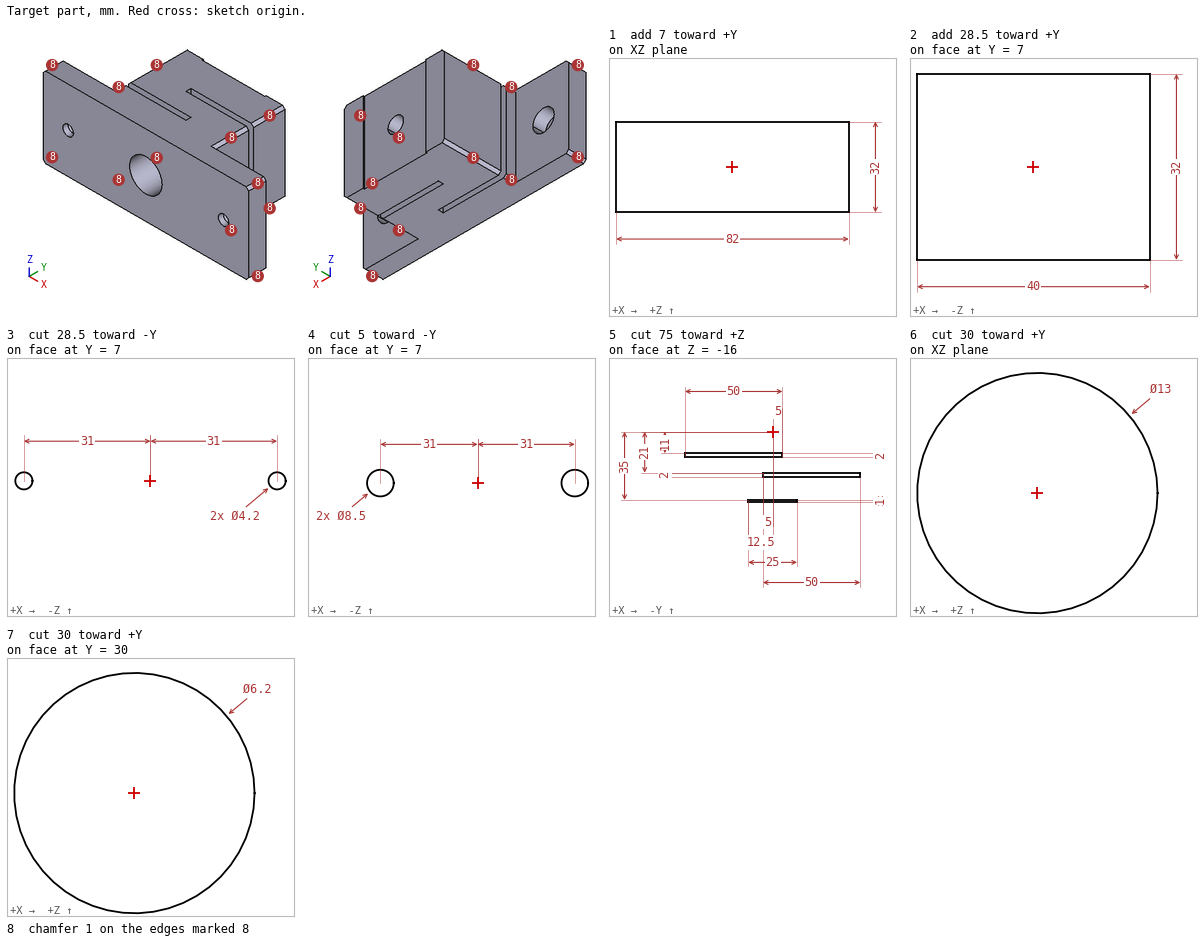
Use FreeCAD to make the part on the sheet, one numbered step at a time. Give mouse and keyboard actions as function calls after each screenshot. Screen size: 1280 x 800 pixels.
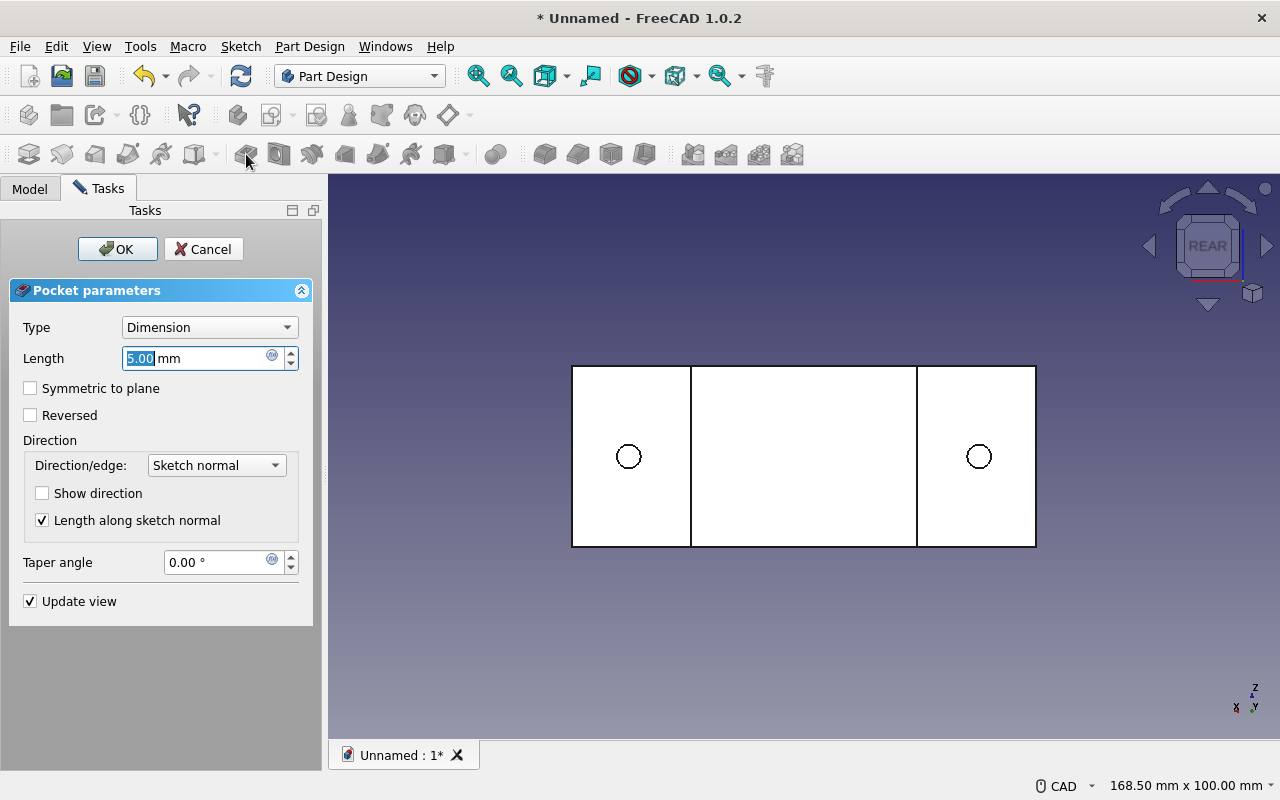
text(28.5)
key(Tab)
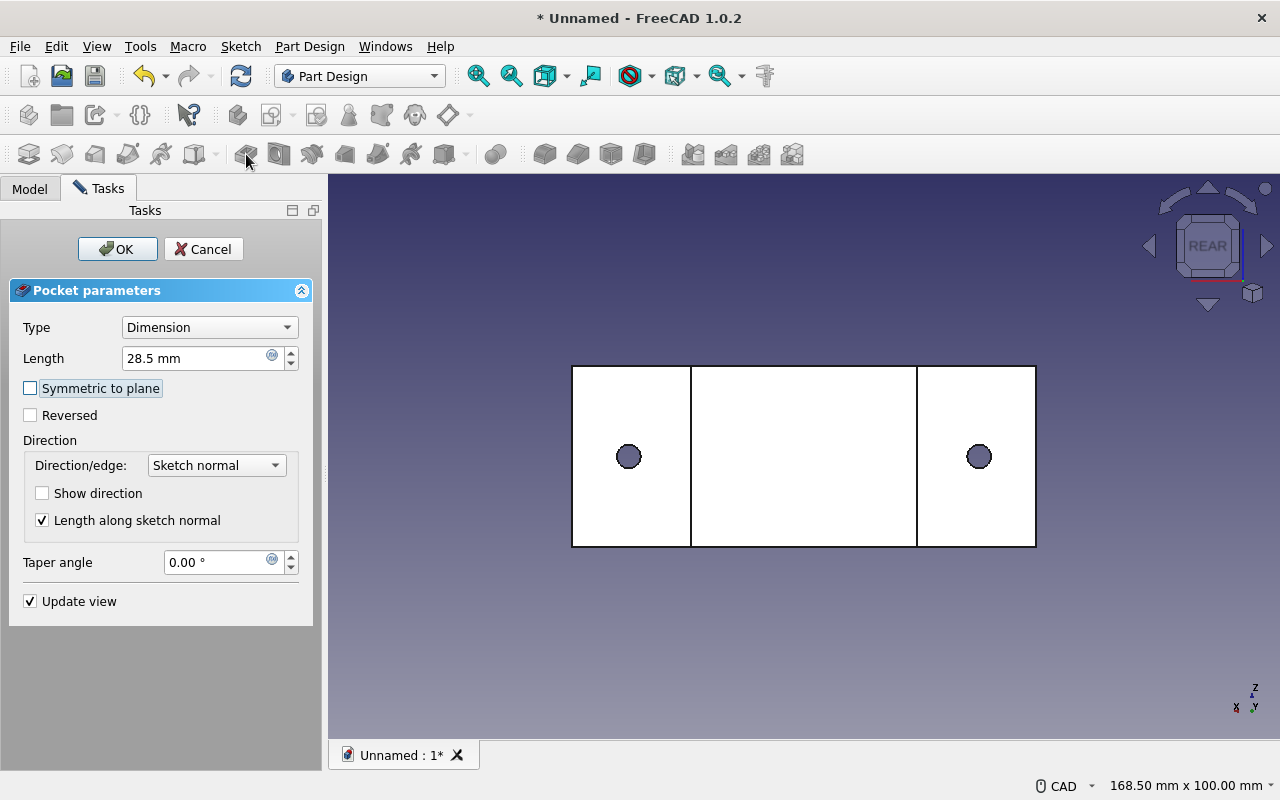
click(118, 249)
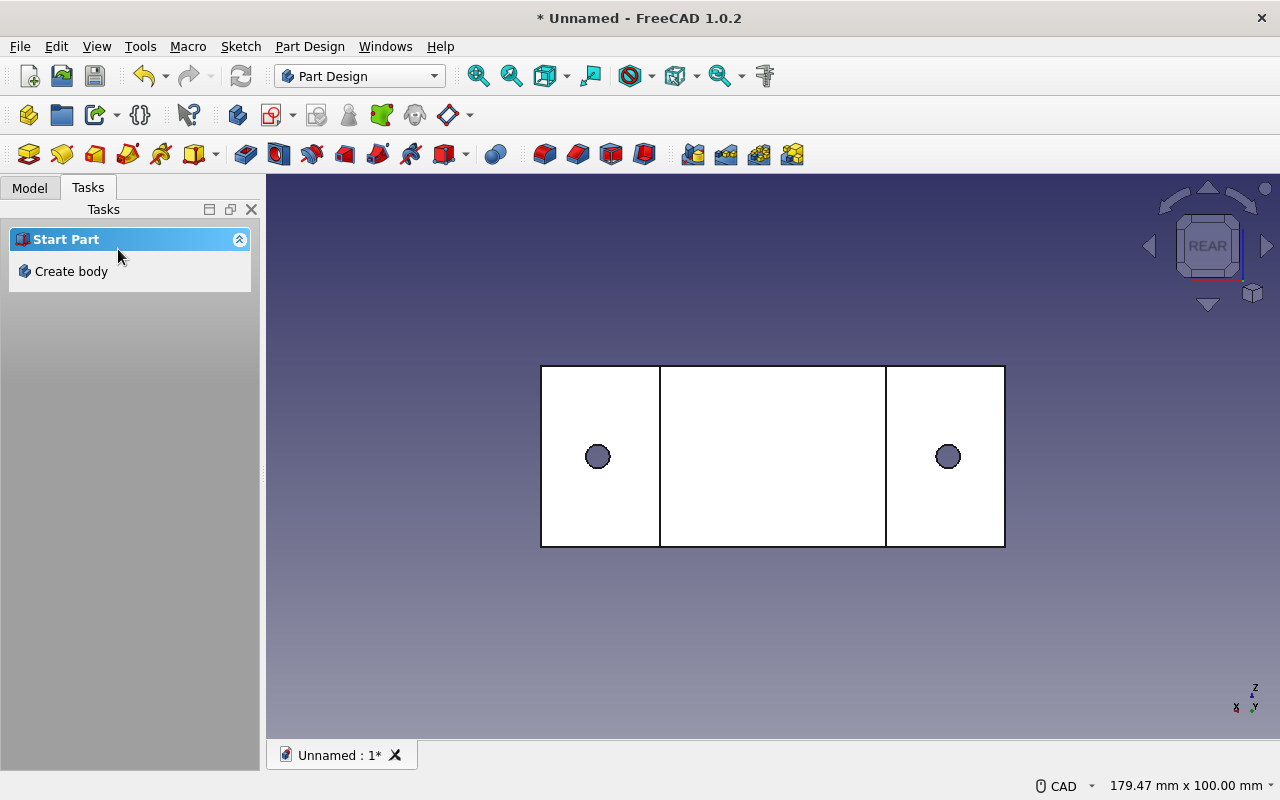
click(584, 404)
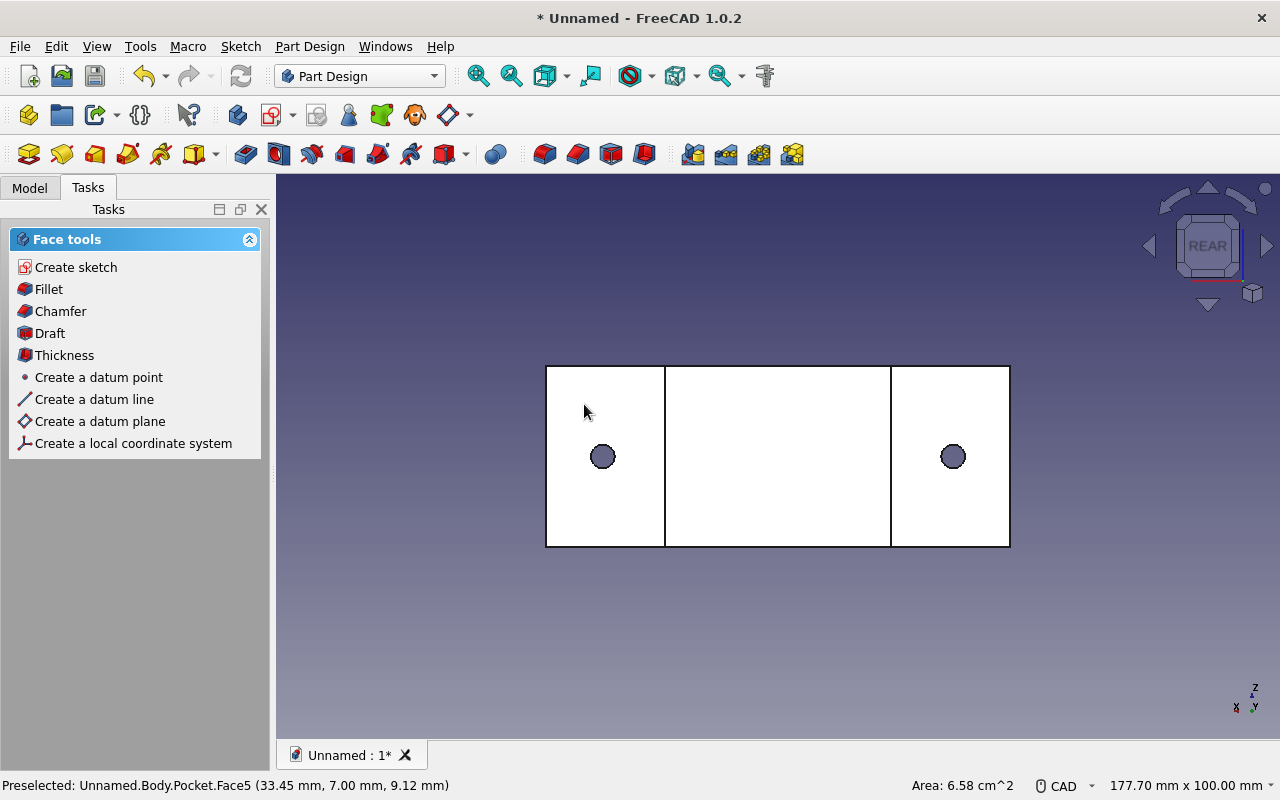
click(270, 116)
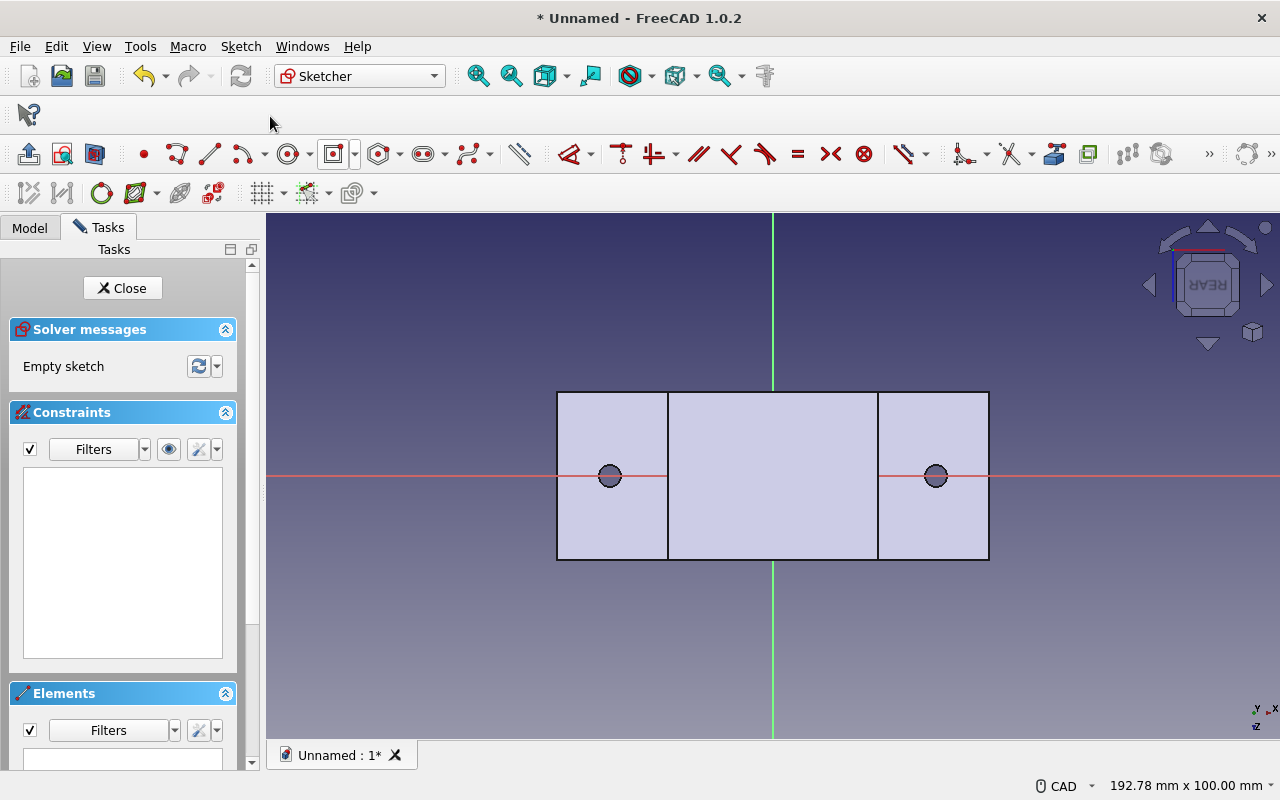
scroll(912, 476, up, 2)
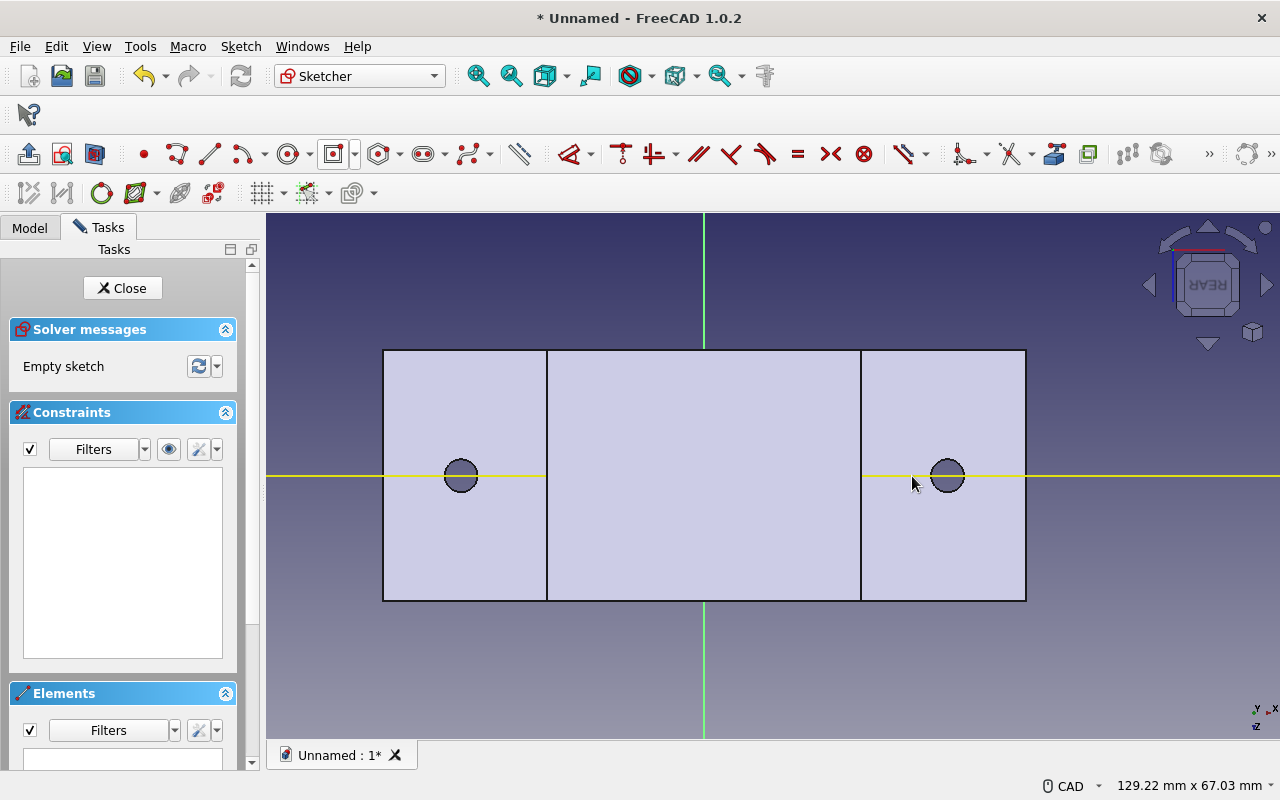
key(g)
key(c)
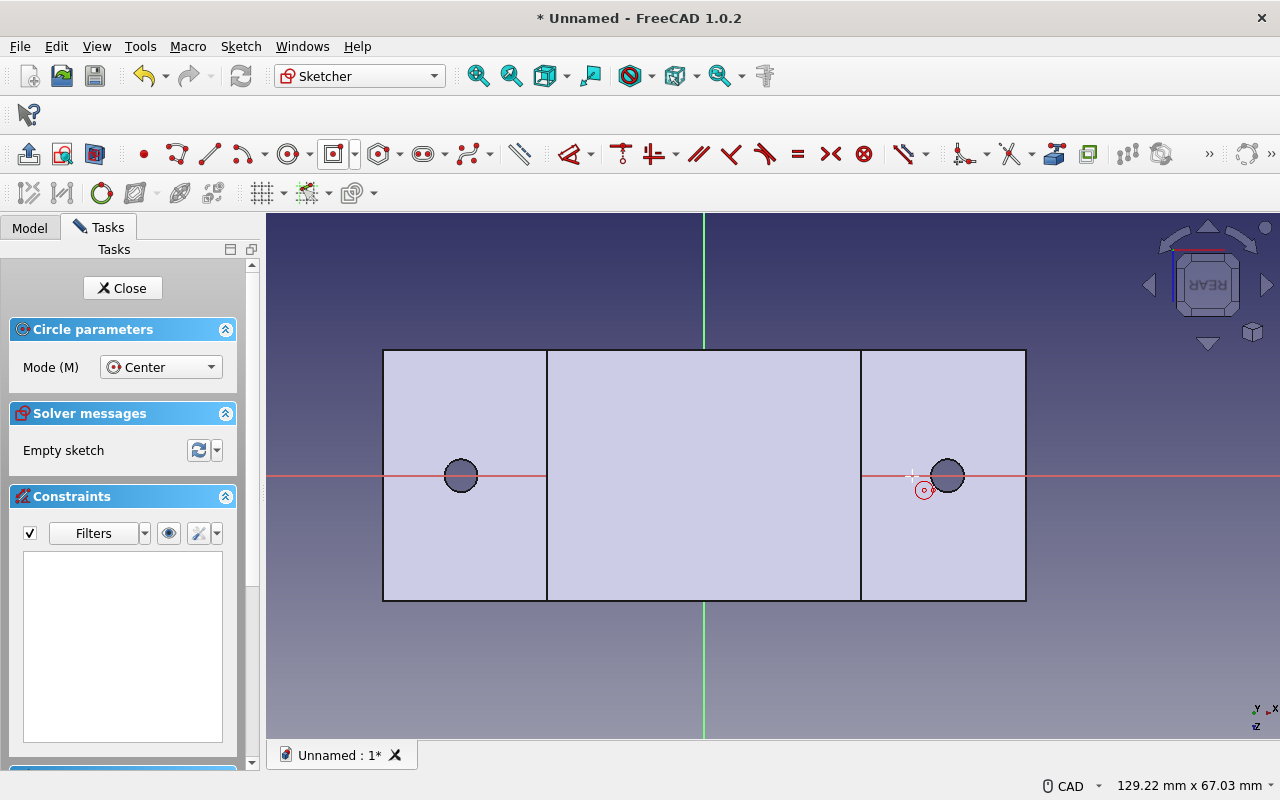
click(461, 476)
move(485, 452)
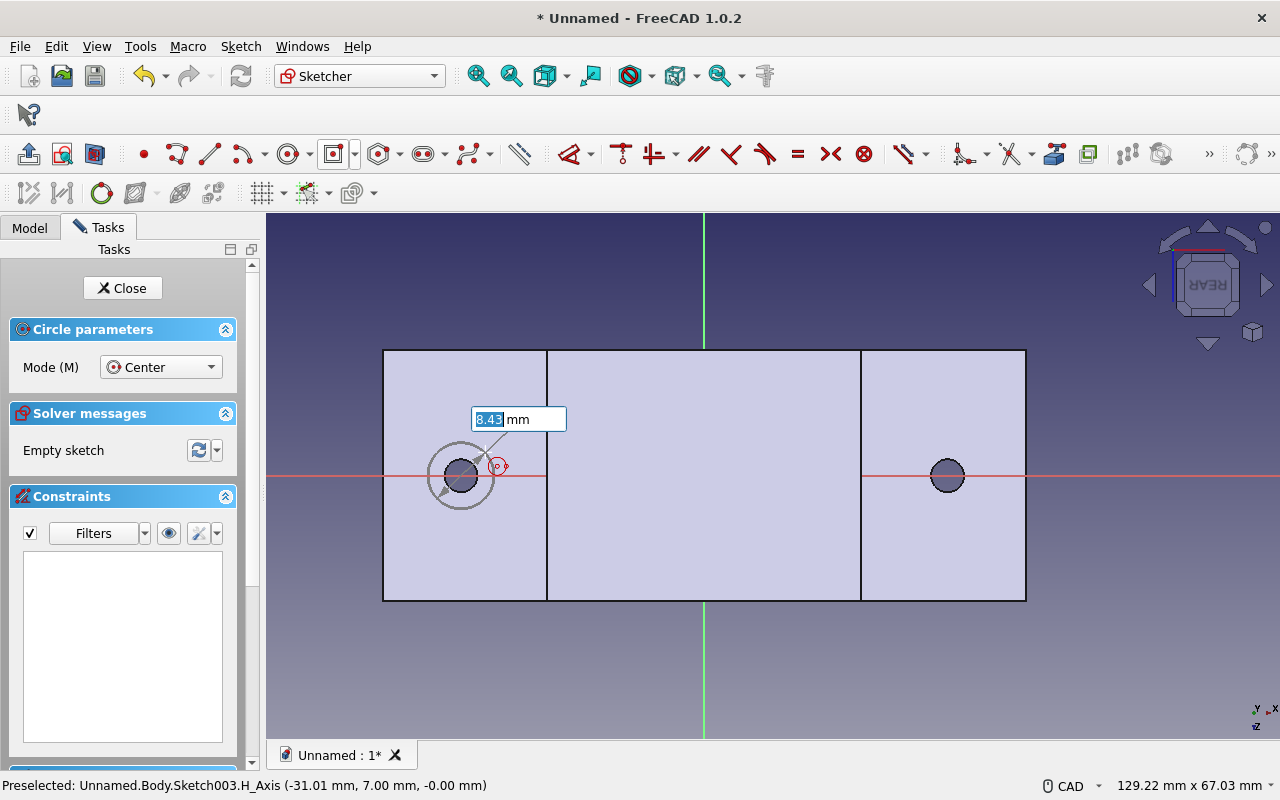
text(8.5)
key(Return)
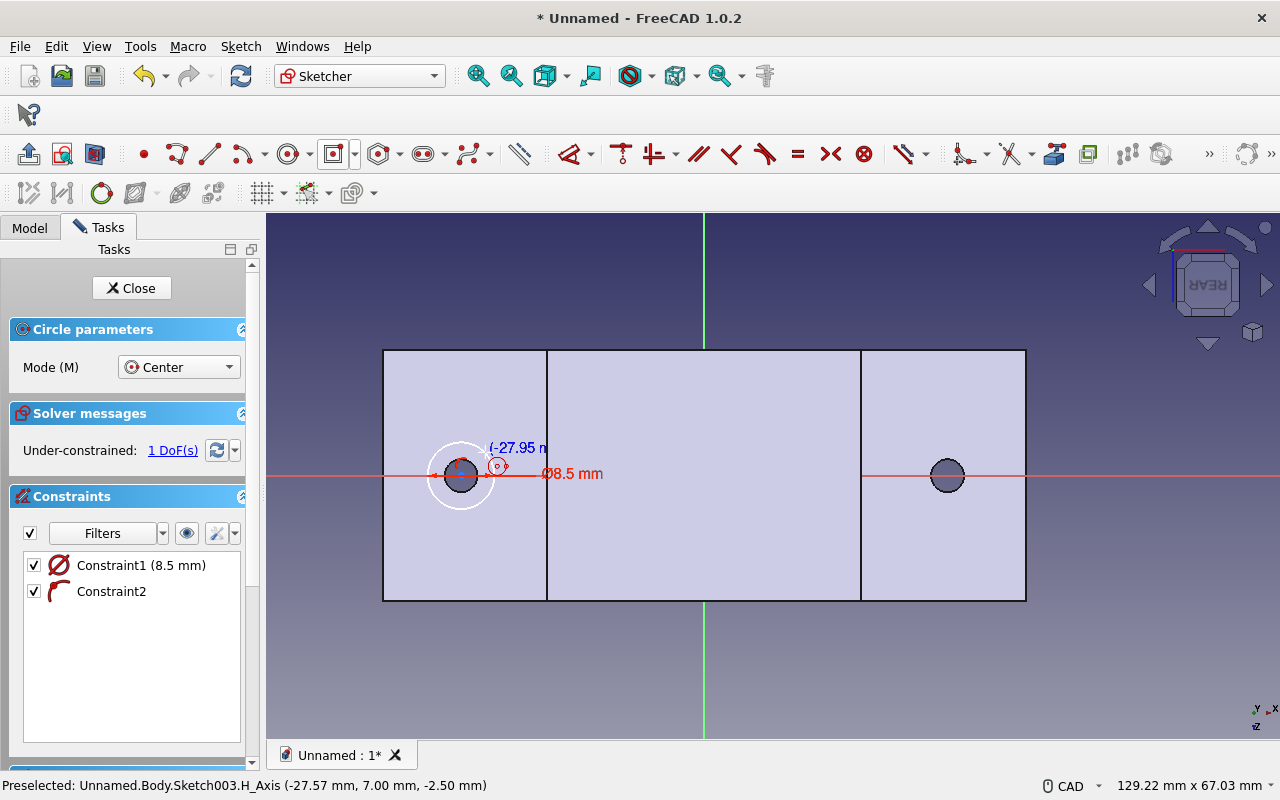
click(948, 476)
move(971, 452)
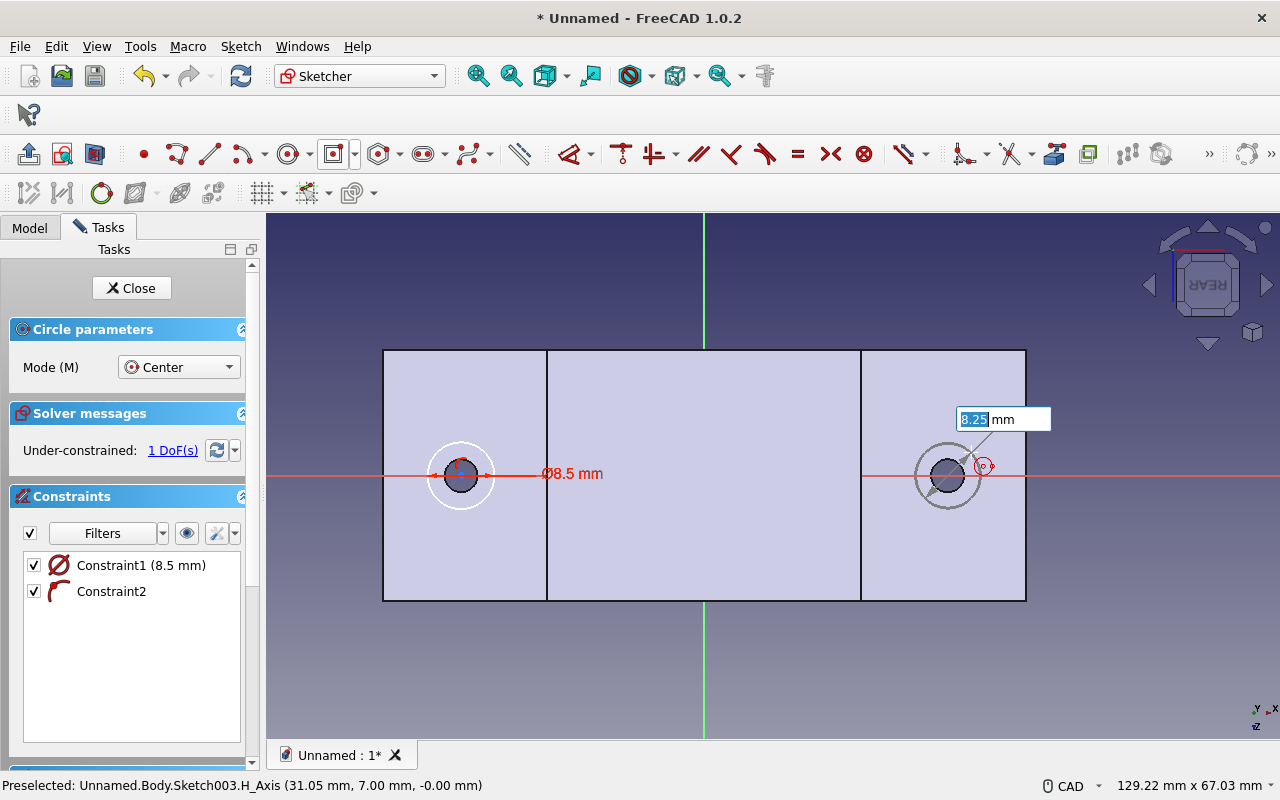
text(8.5)
key(Return)
key(Escape)